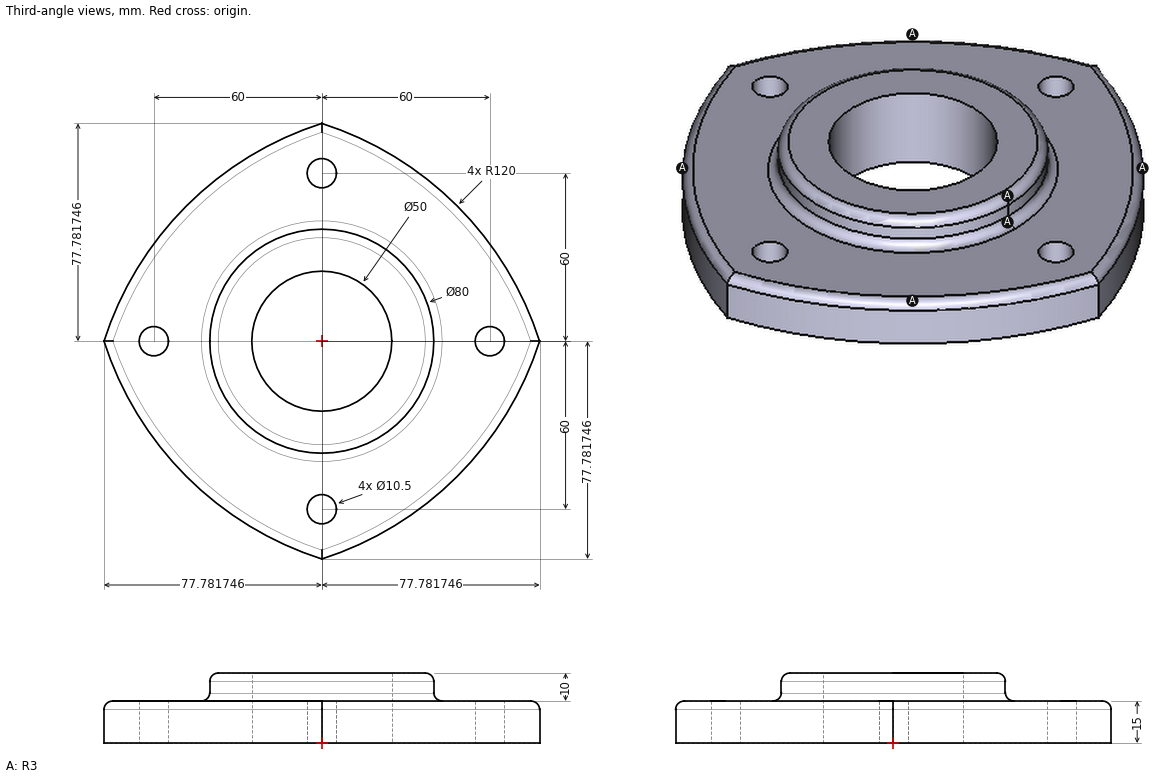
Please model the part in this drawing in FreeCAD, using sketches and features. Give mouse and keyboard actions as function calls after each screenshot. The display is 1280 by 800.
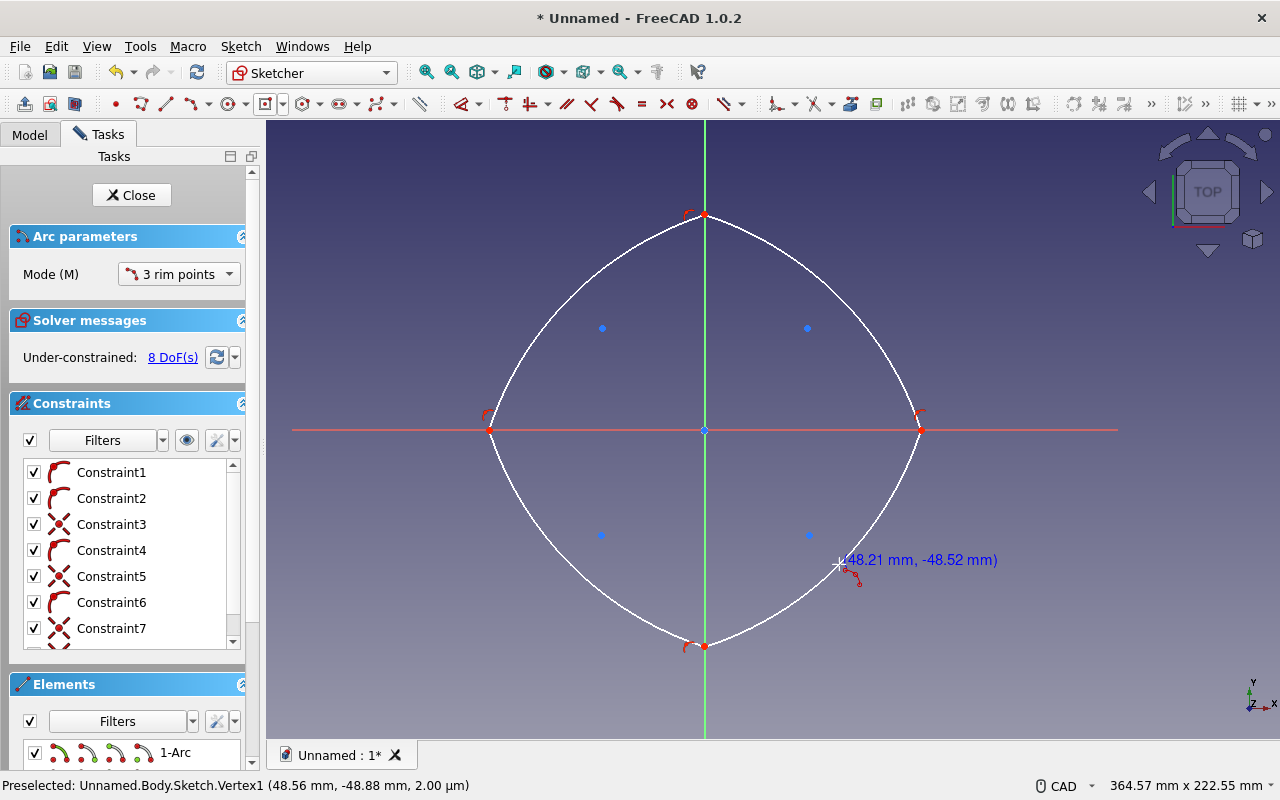
key(g)
key(c)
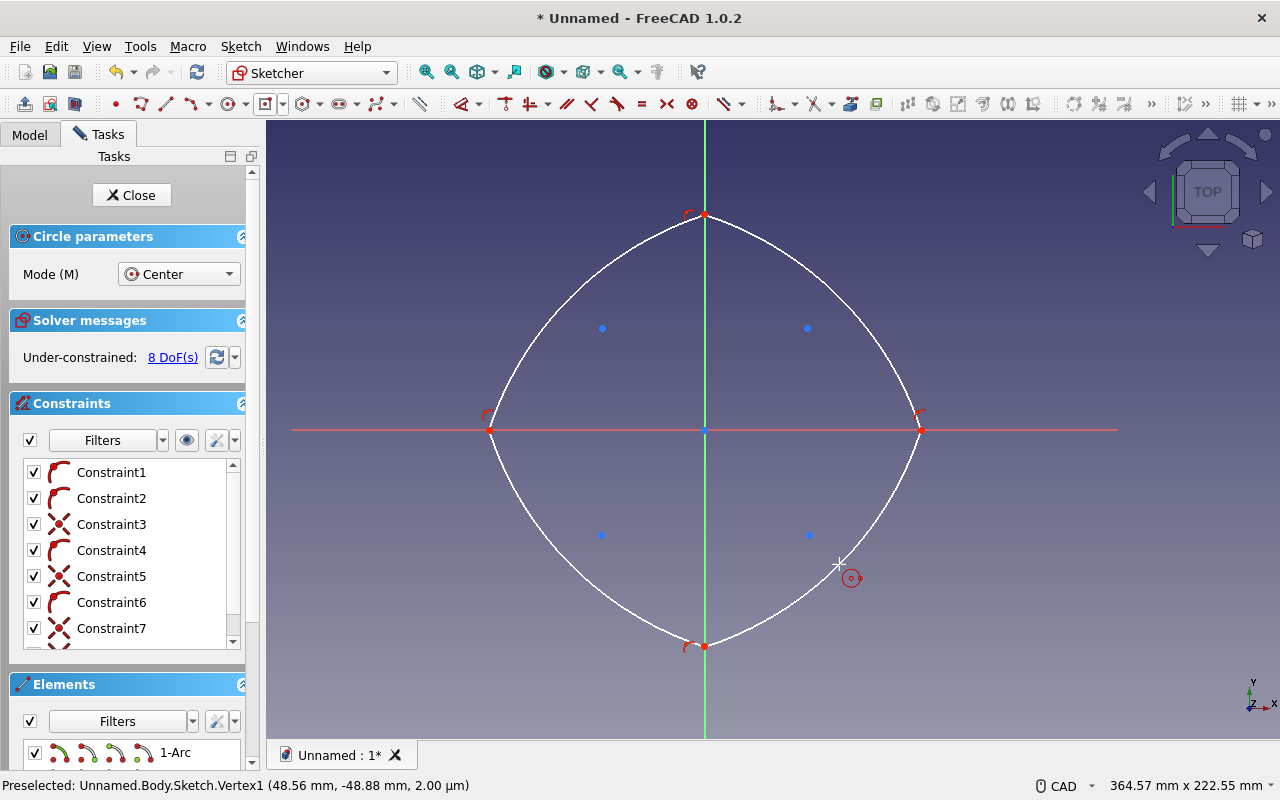
scroll(705, 597, up, 3)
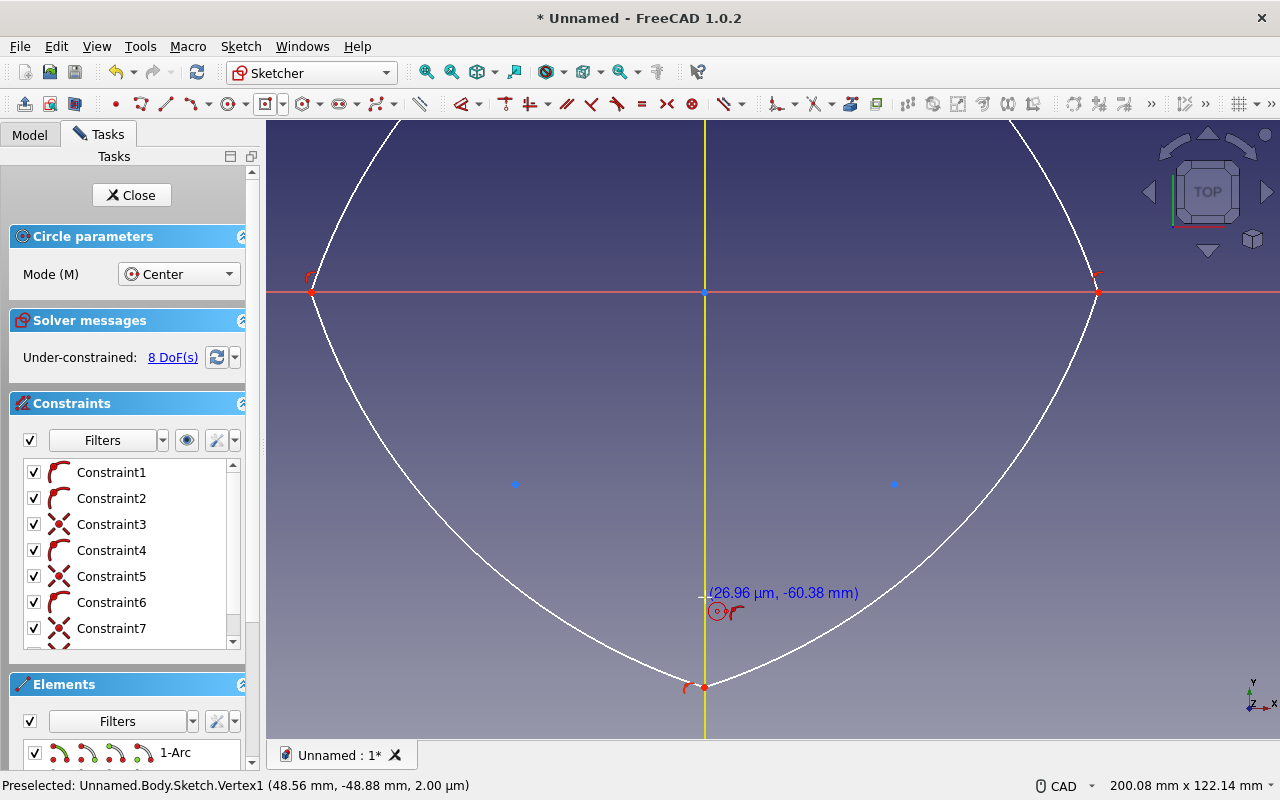
click(705, 596)
click(723, 577)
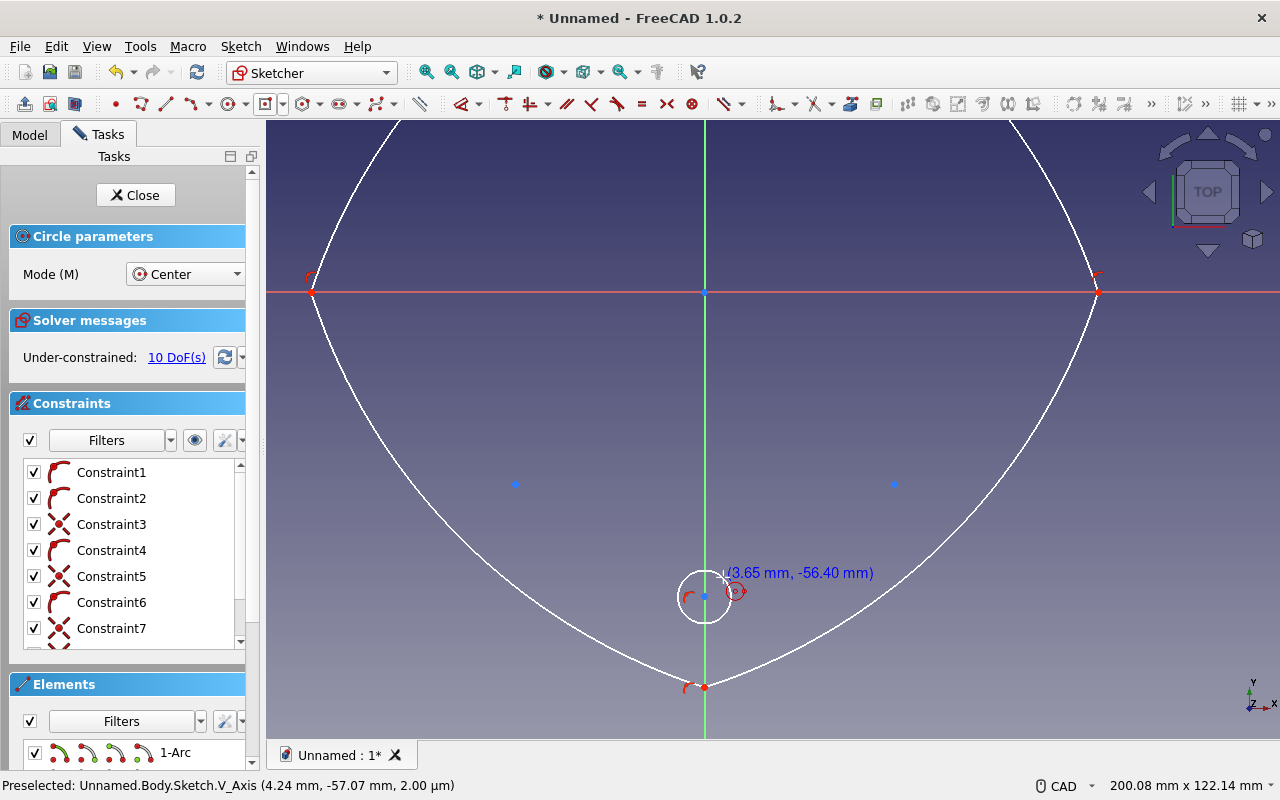
click(1009, 292)
click(1027, 273)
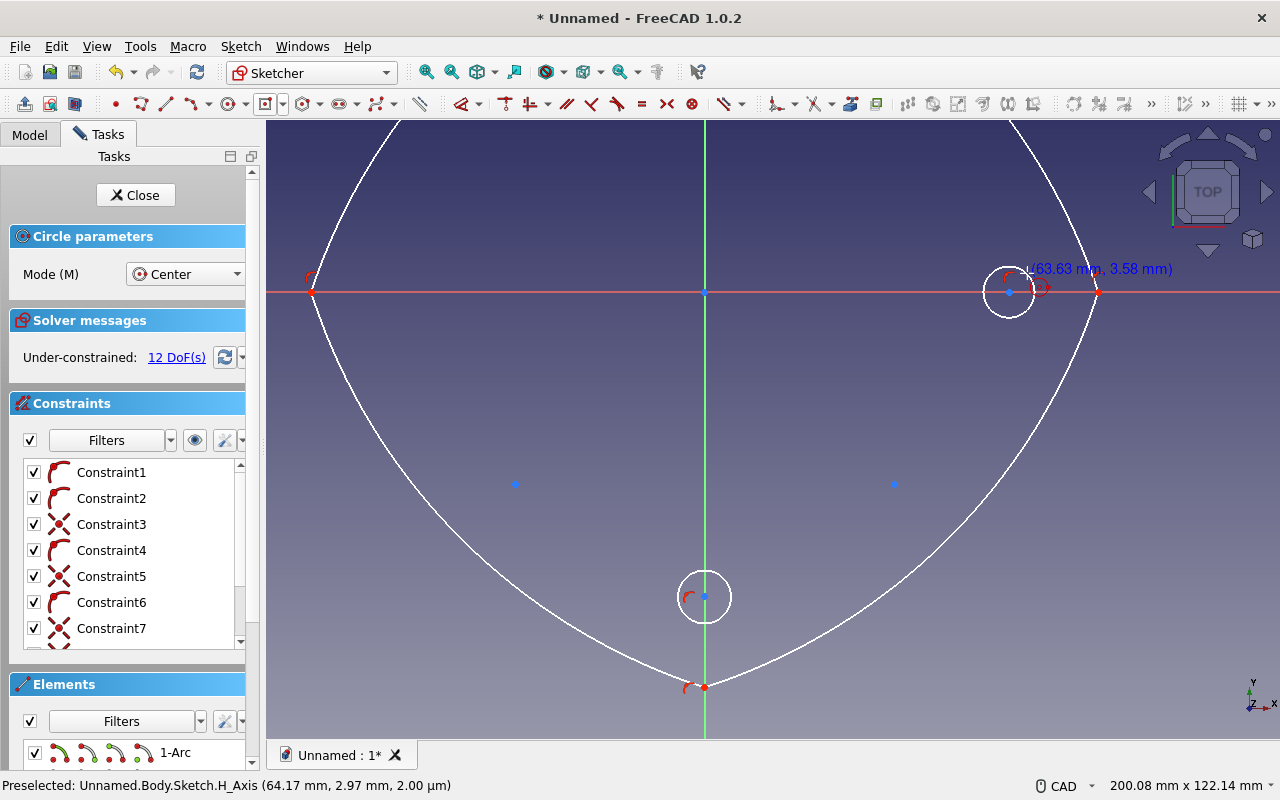
click(400, 292)
click(419, 273)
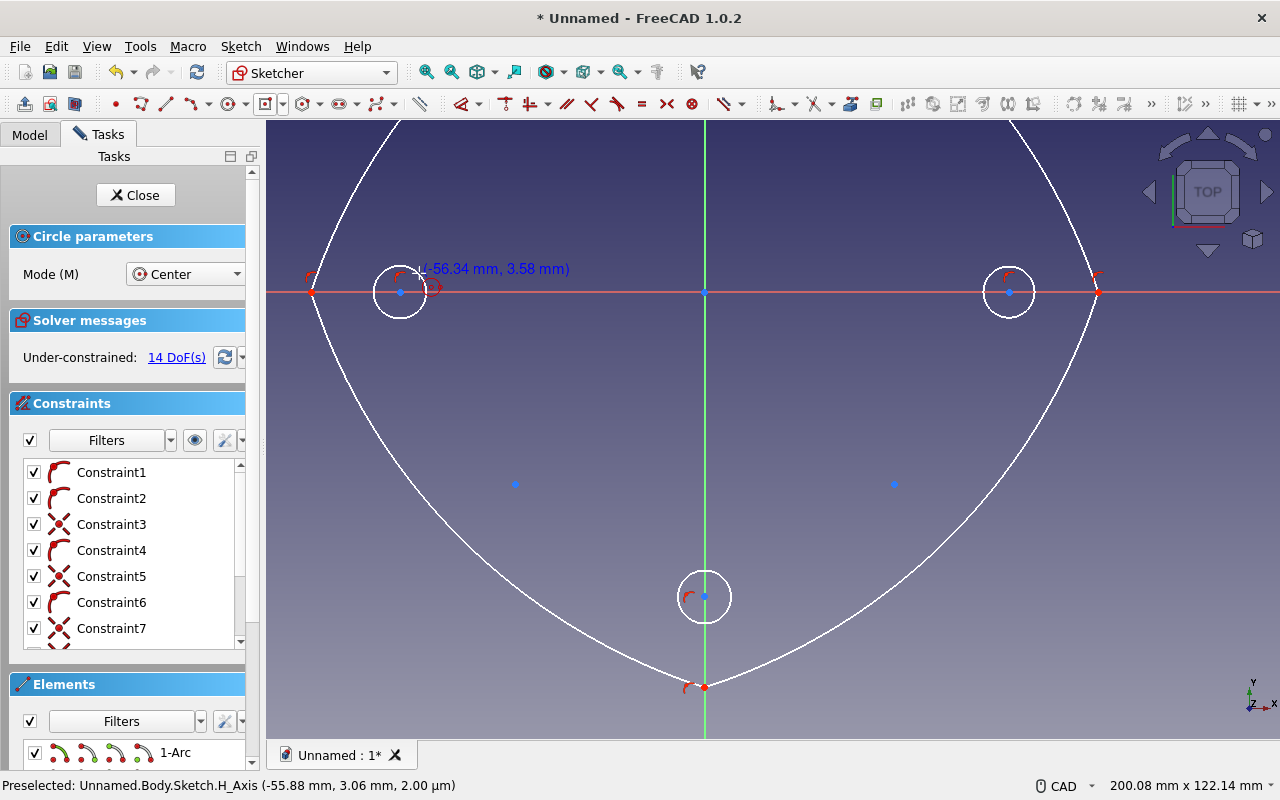
scroll(704, 597, down, 3)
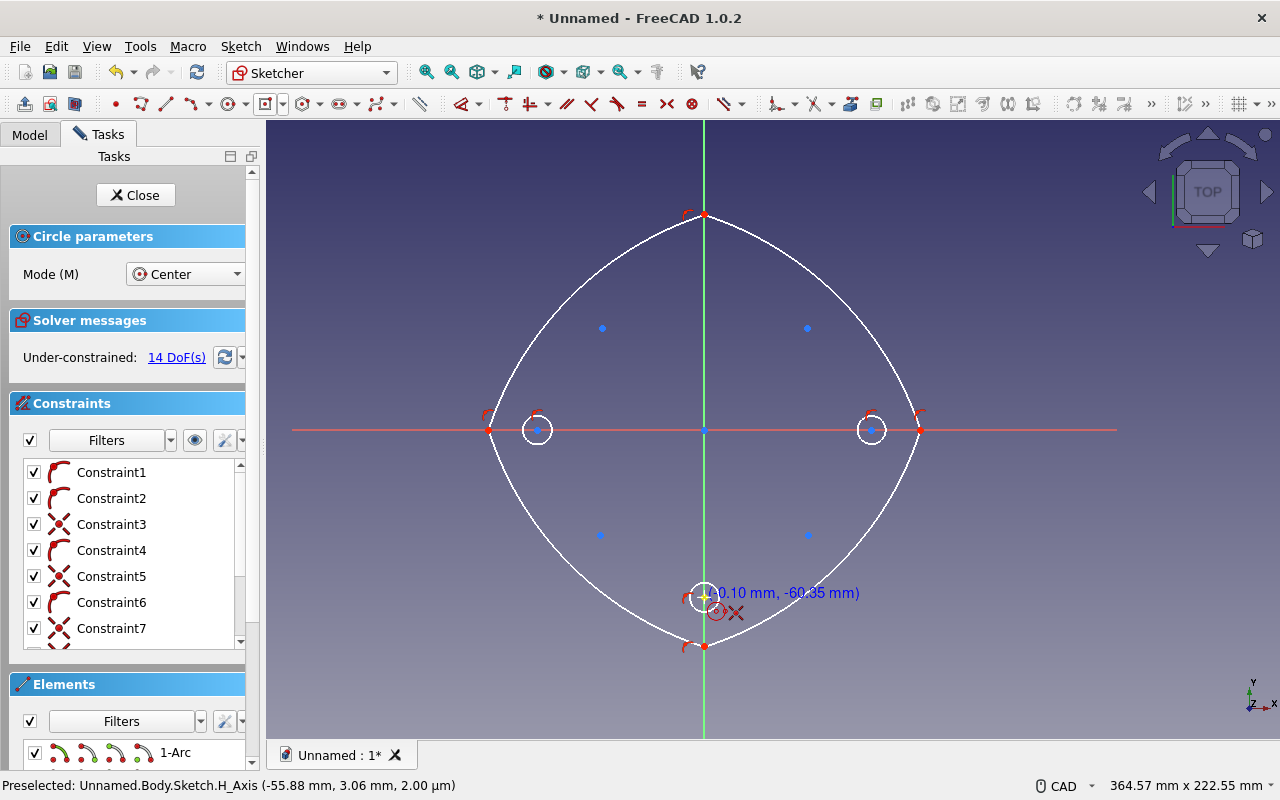
scroll(704, 263, up, 3)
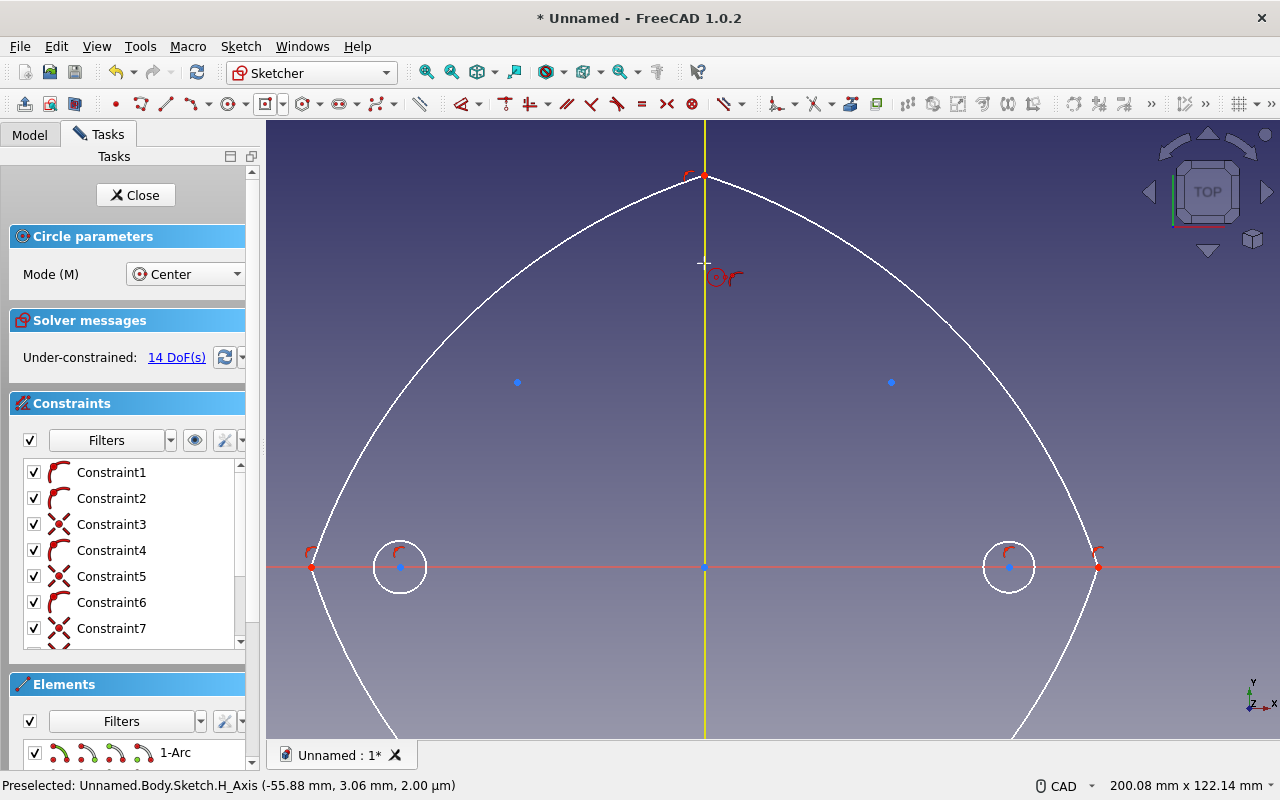
click(705, 263)
click(723, 244)
key(Escape)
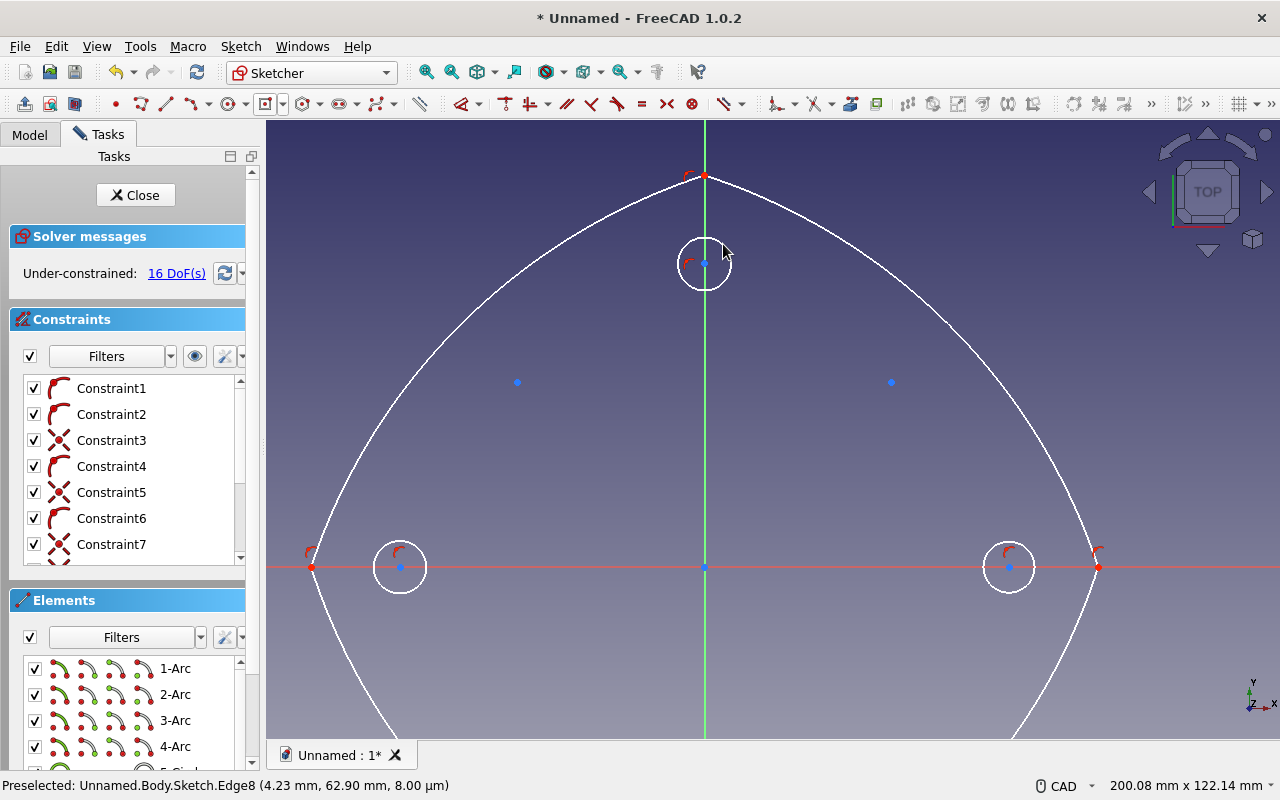
click(1022, 413)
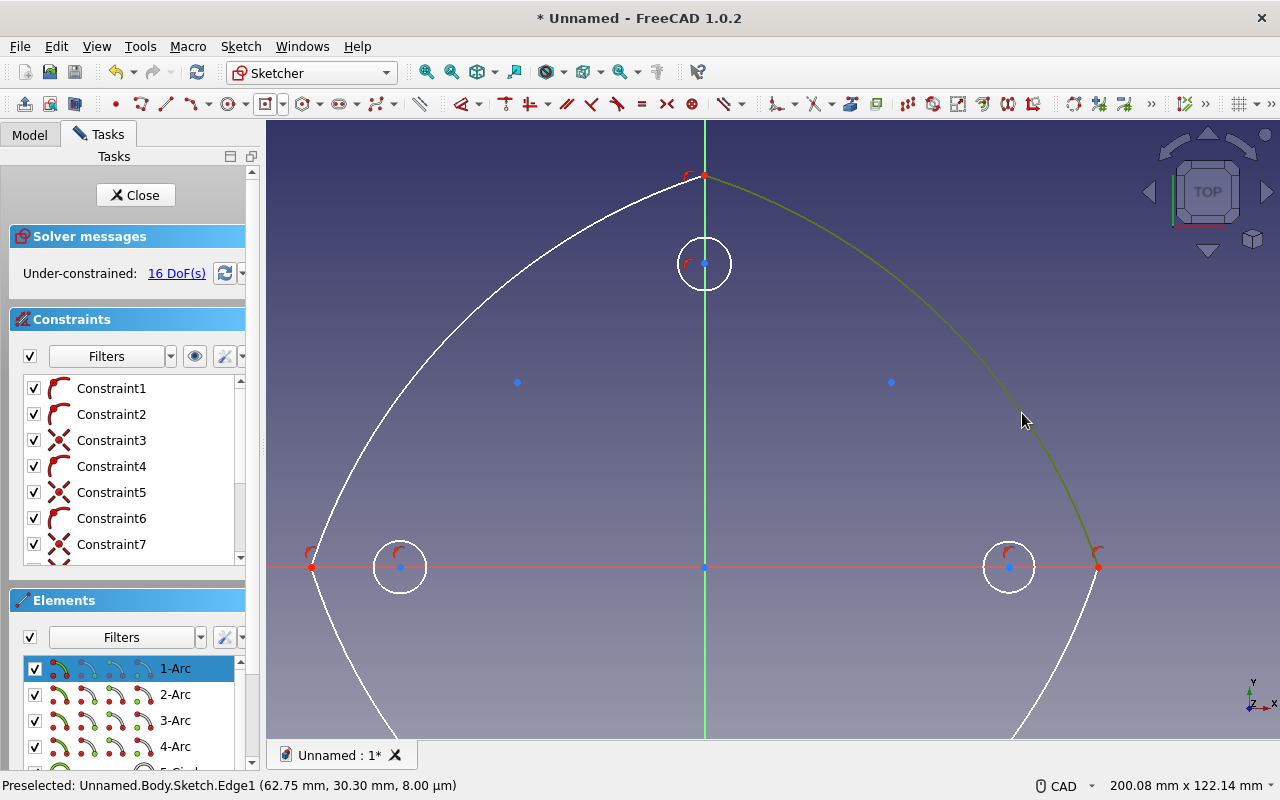
click(550, 251)